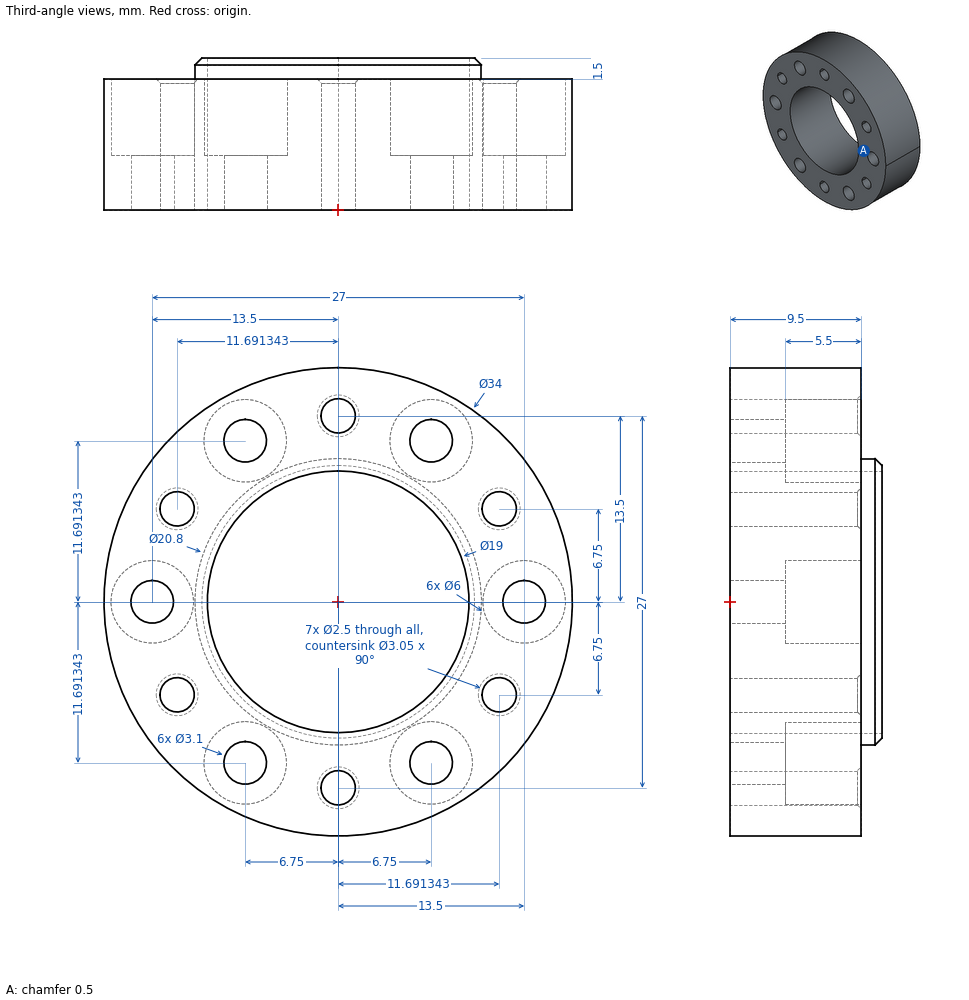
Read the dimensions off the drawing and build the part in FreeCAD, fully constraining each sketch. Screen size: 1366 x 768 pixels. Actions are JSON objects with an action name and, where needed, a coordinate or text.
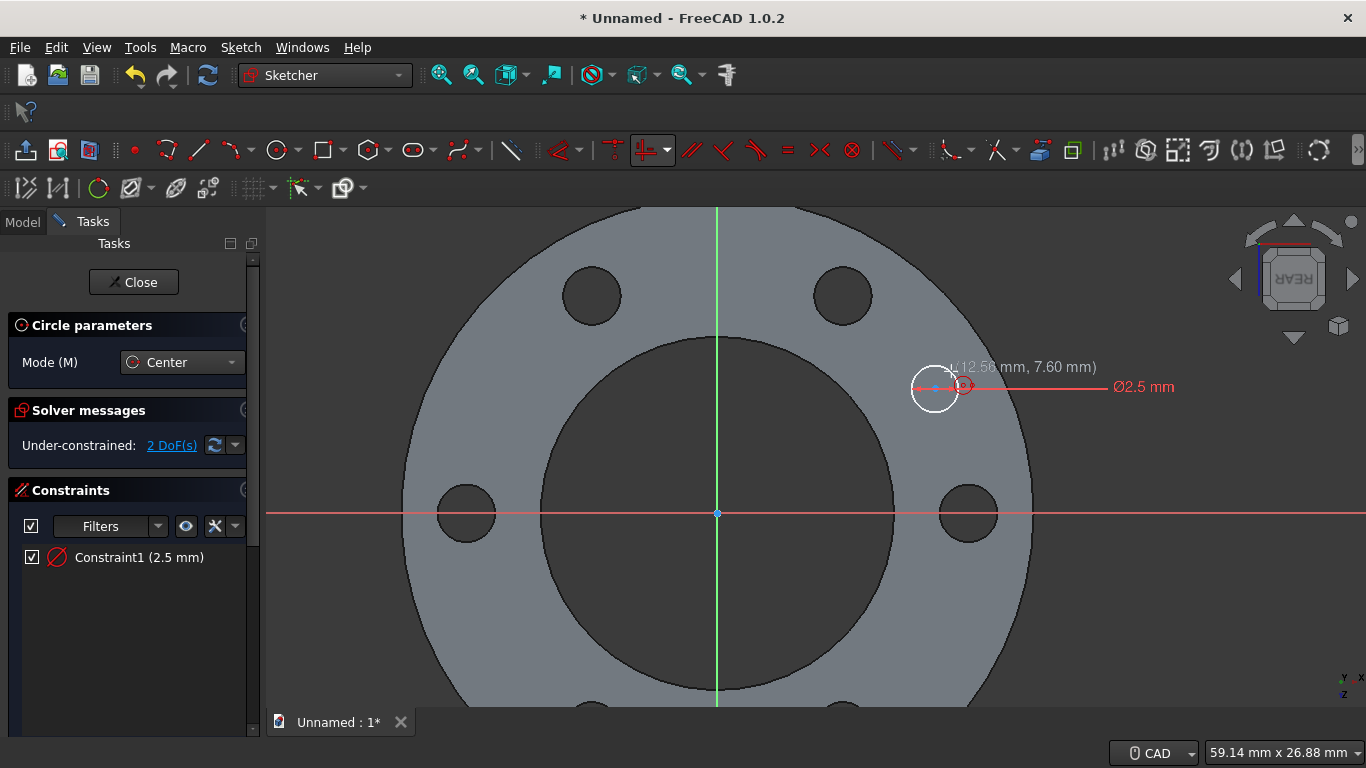
{"action": "left_click", "coordinate": [935, 639]}
{"action": "mouse_move", "coordinate": [951, 623]}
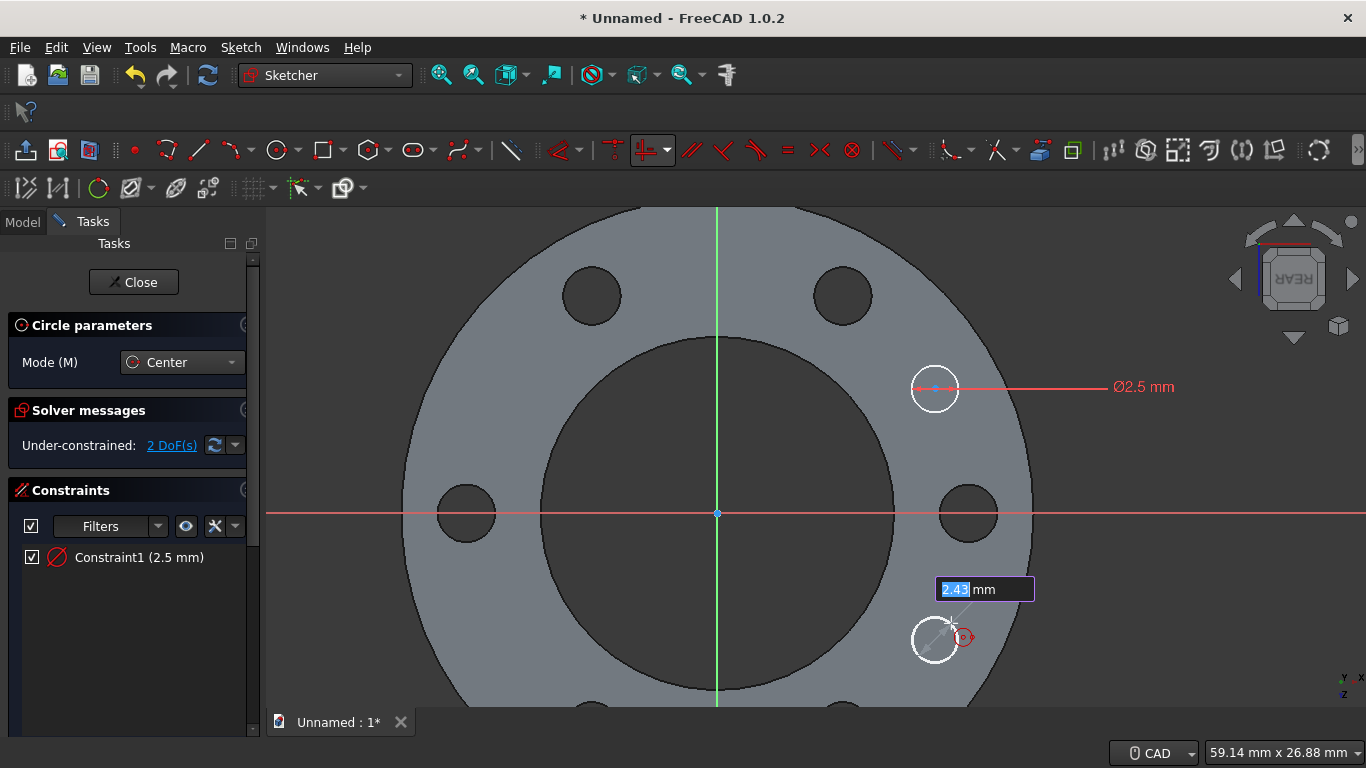
{"action": "type", "text": "2.5"}
{"action": "key", "text": "Return"}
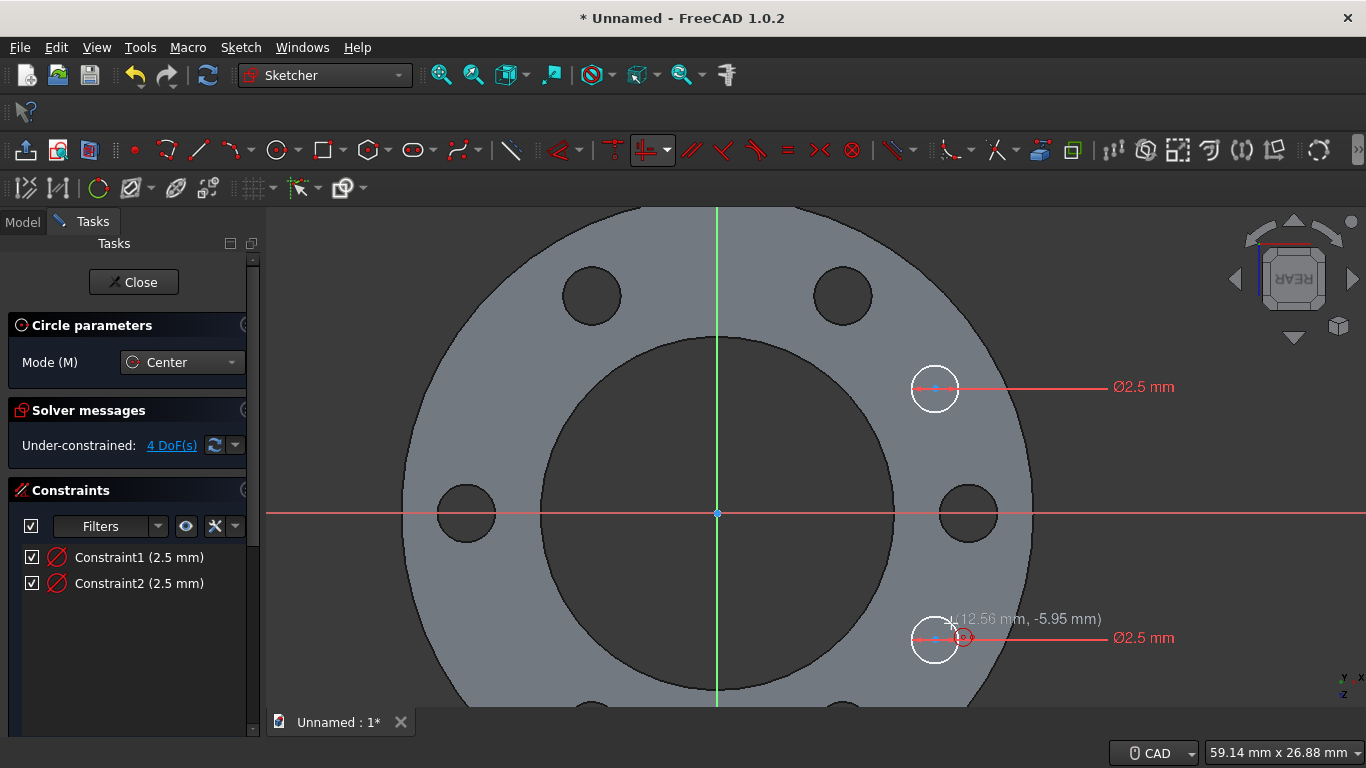
{"action": "scroll", "coordinate": [784, 388], "scroll_direction": "down", "scroll_amount": 3}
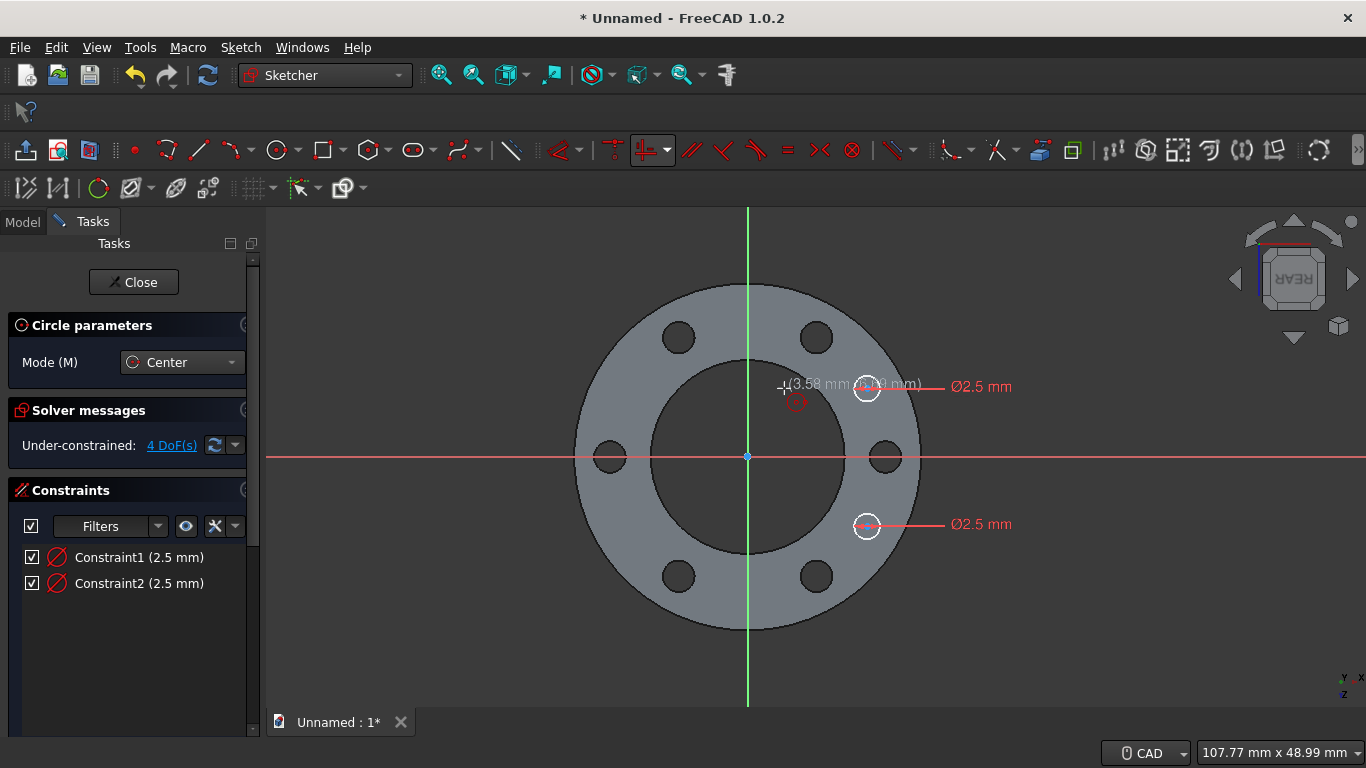
{"action": "scroll", "coordinate": [748, 595], "scroll_direction": "up", "scroll_amount": 3}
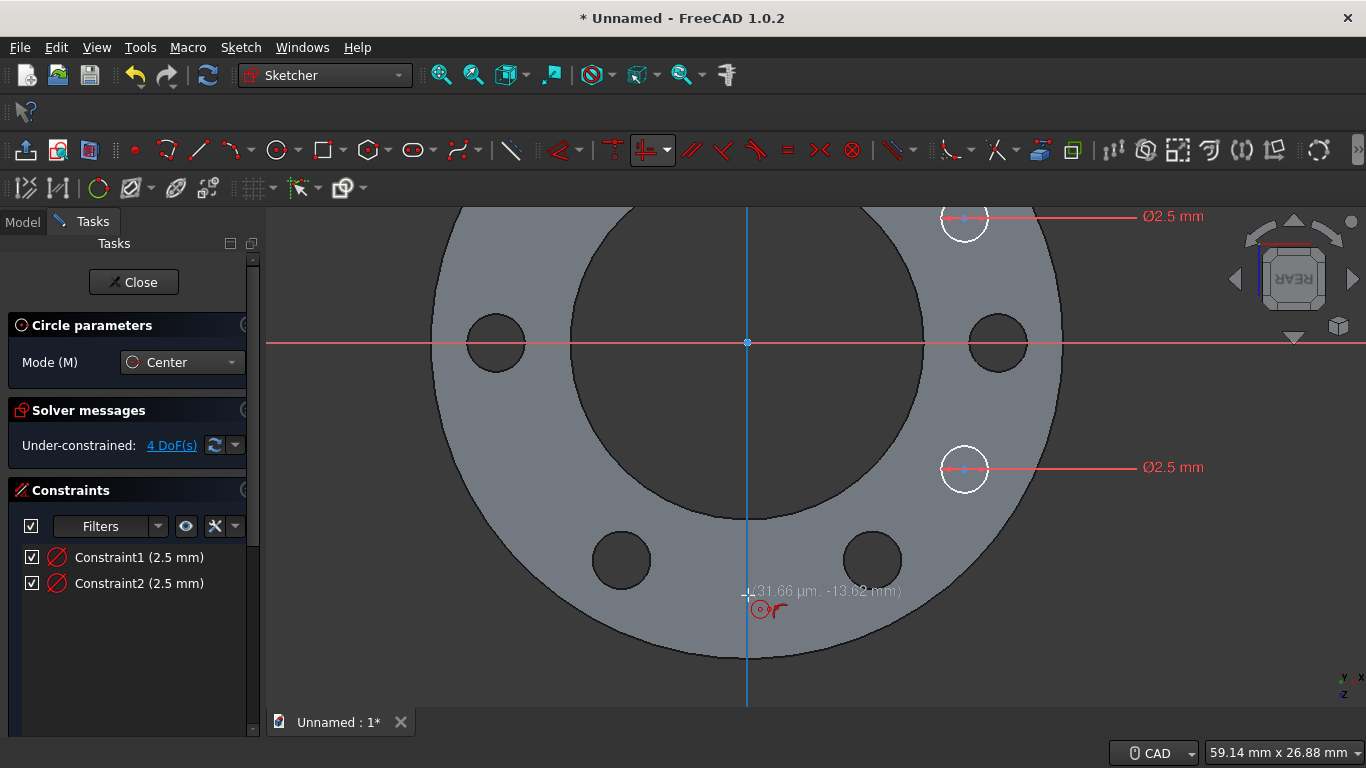
{"action": "left_click", "coordinate": [747, 594]}
{"action": "mouse_move", "coordinate": [763, 578]}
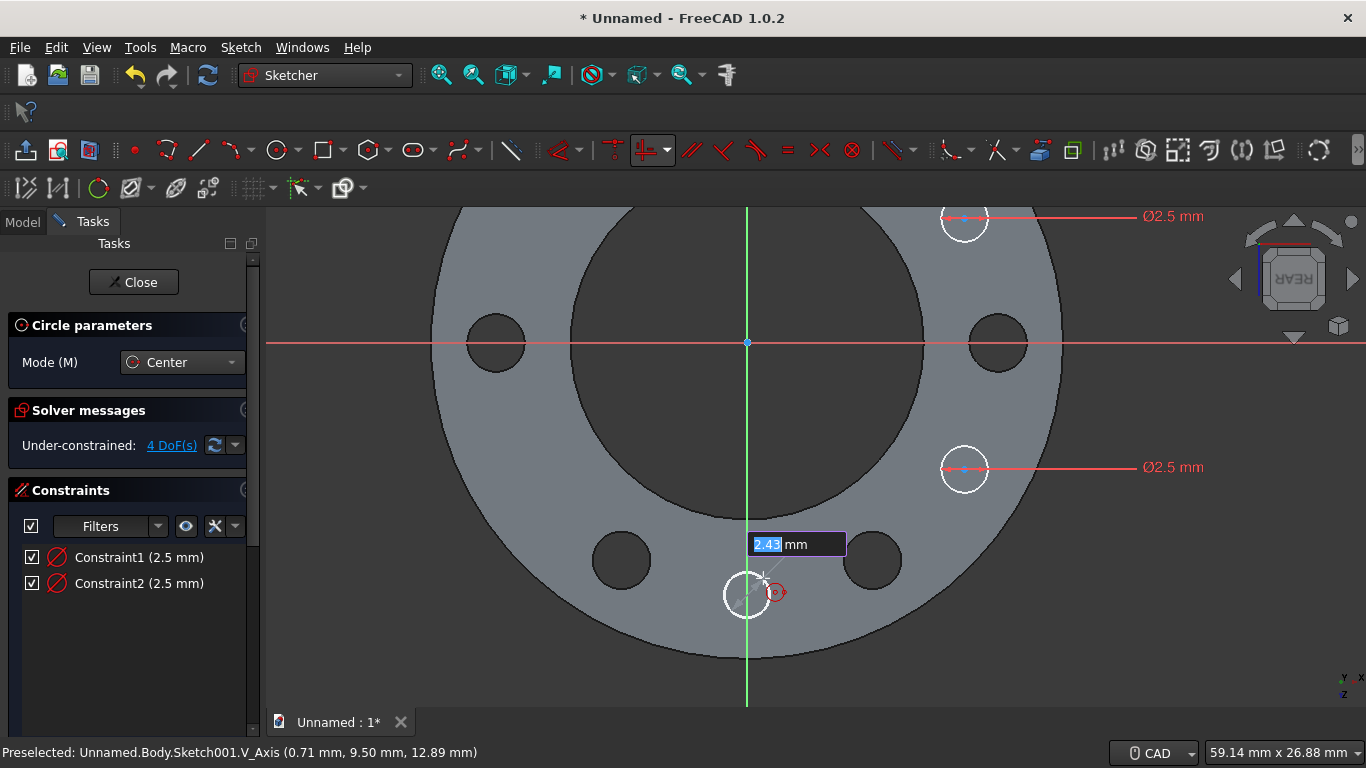
{"action": "type", "text": "2.5"}
{"action": "key", "text": "Return"}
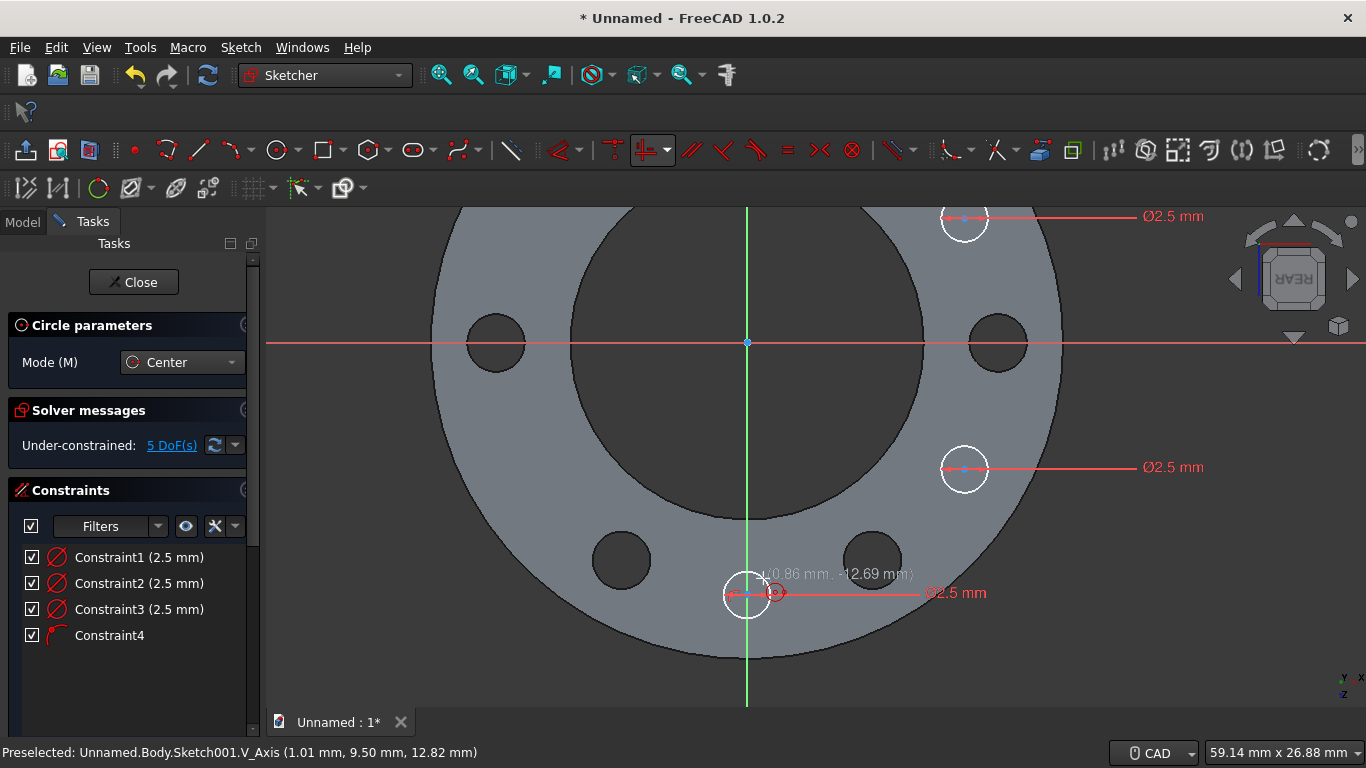
{"action": "left_click", "coordinate": [530, 468]}
{"action": "mouse_move", "coordinate": [546, 452]}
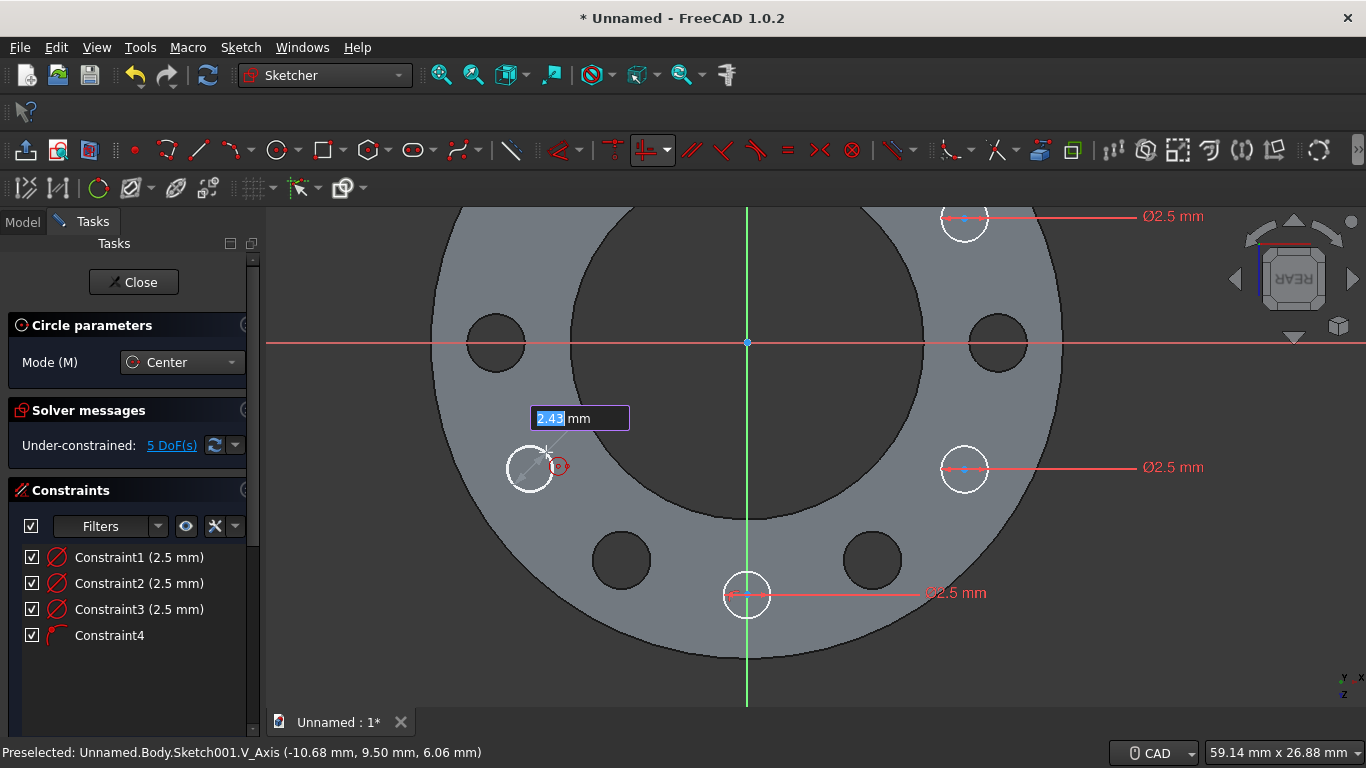
{"action": "type", "text": "2.5"}
{"action": "key", "text": "Return"}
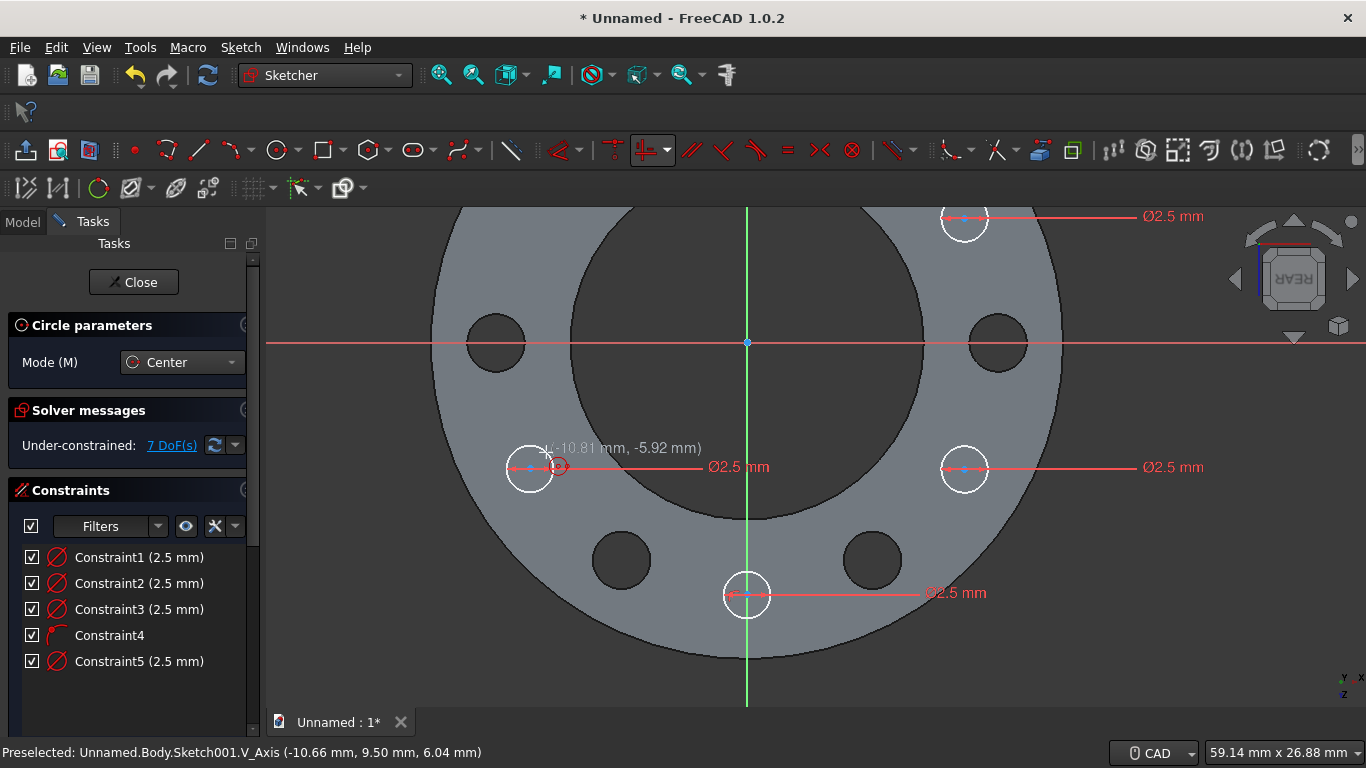
{"action": "scroll", "coordinate": [748, 596], "scroll_direction": "down", "scroll_amount": 3}